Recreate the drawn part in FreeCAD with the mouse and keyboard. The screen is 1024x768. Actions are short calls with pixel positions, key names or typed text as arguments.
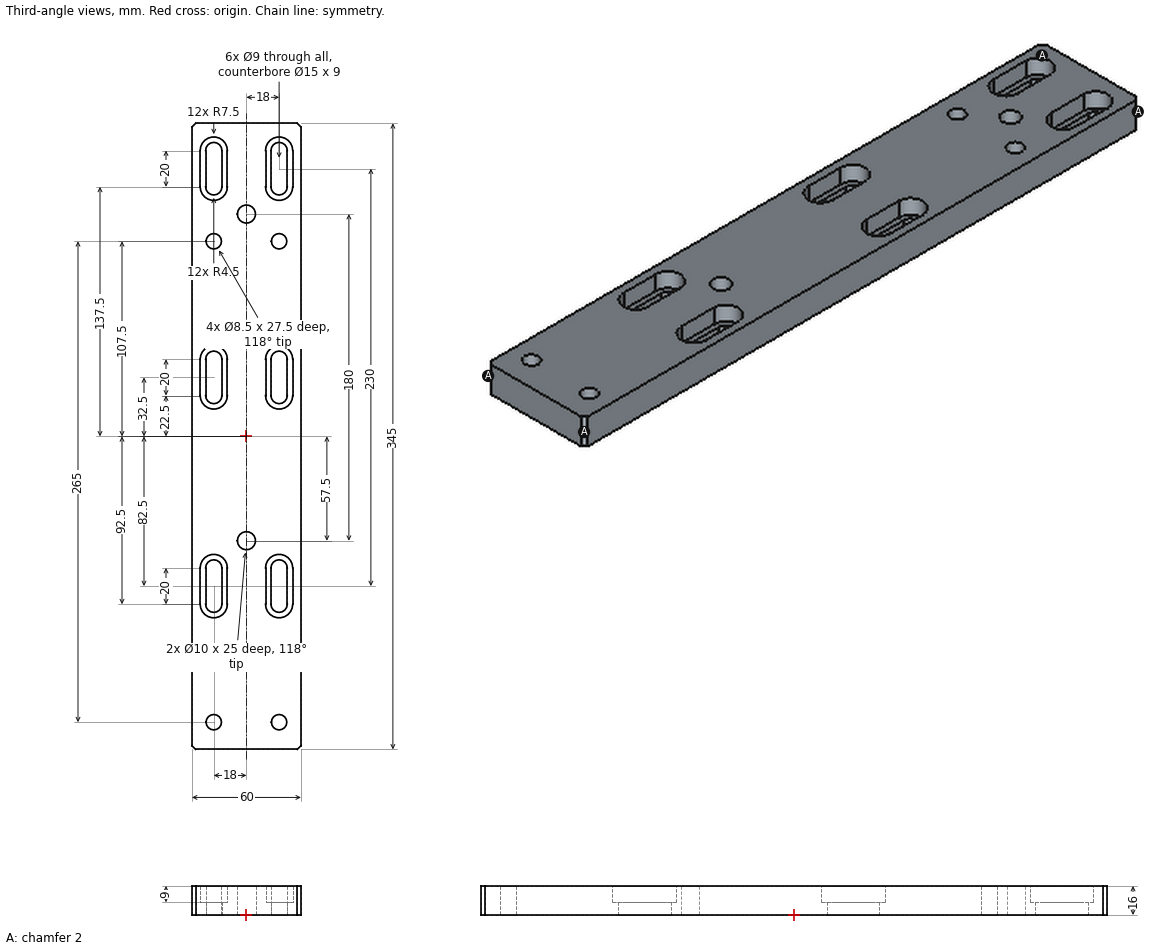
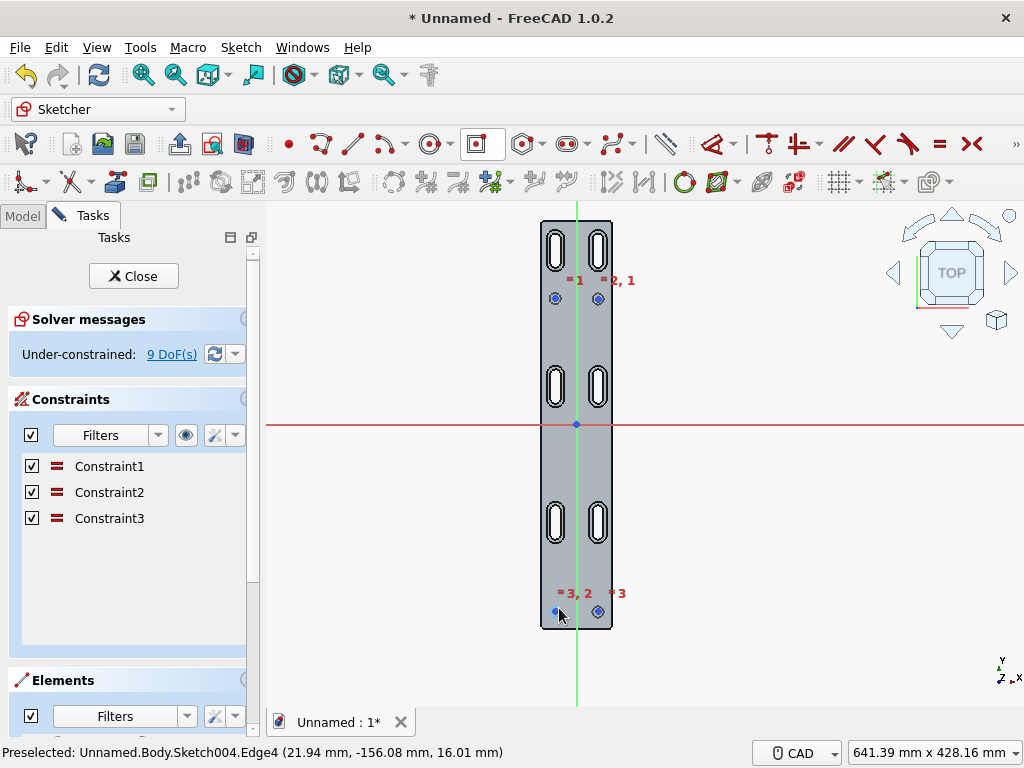
click(555, 299)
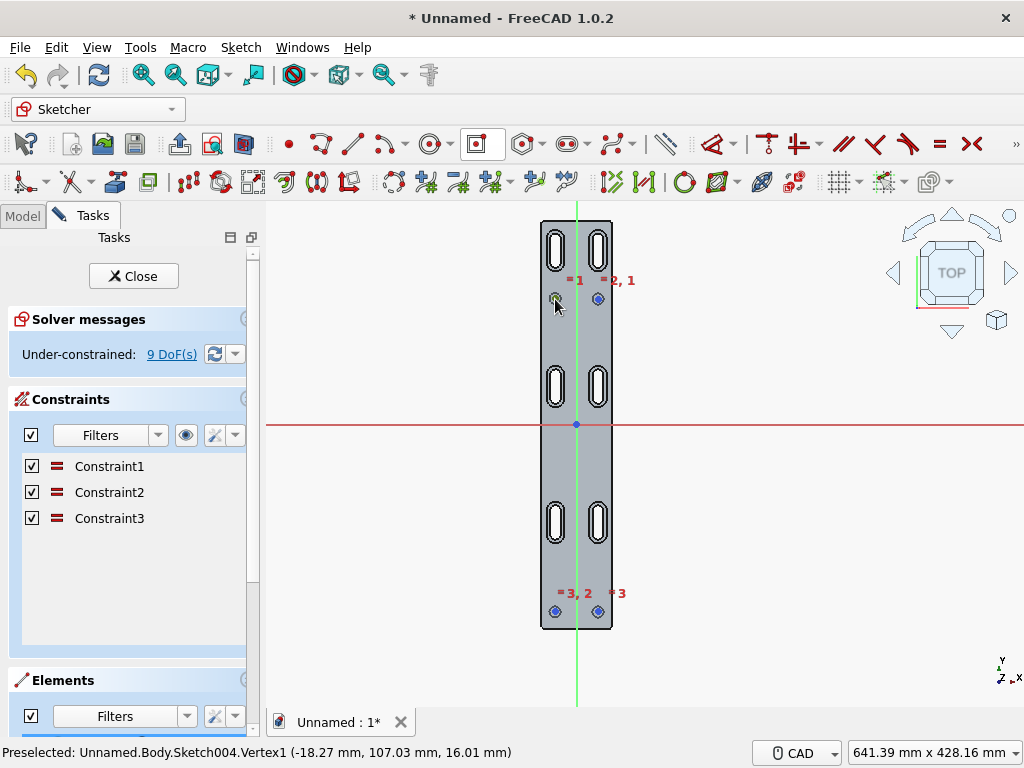
click(598, 299)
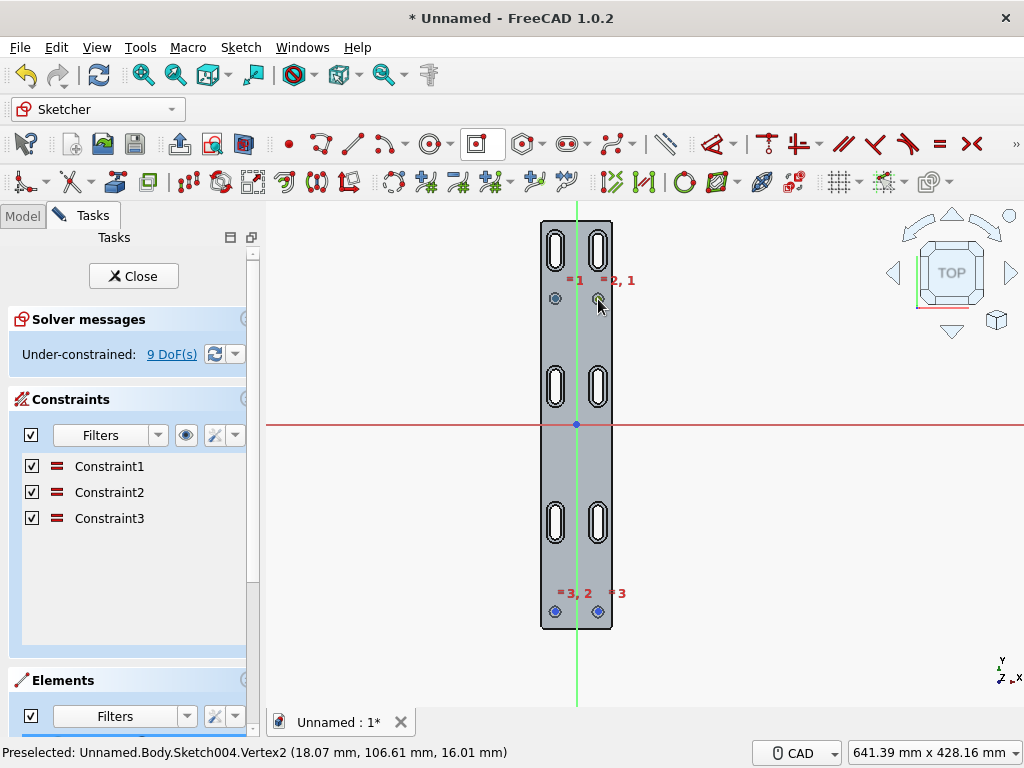
click(577, 647)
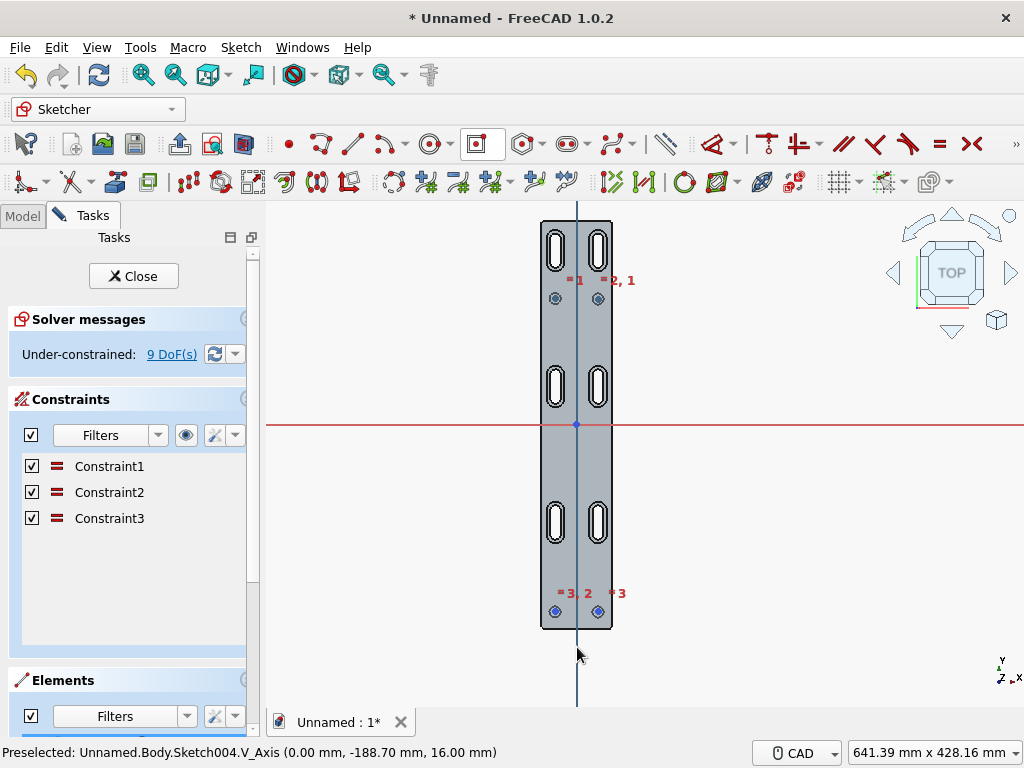
key(s)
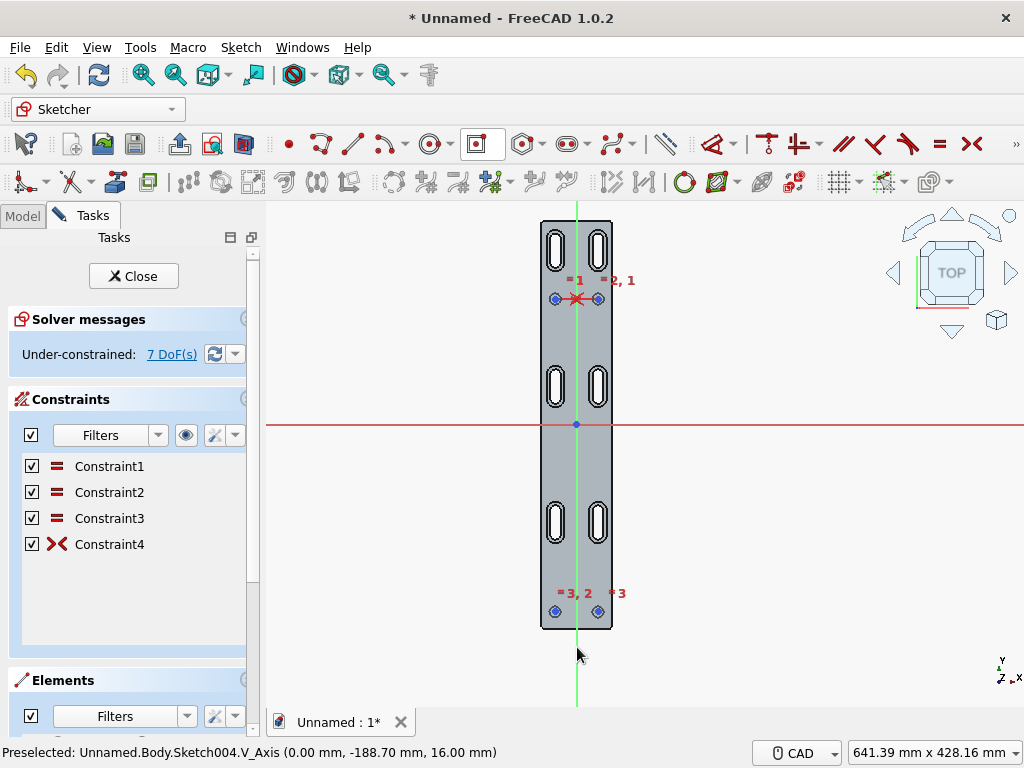
click(555, 612)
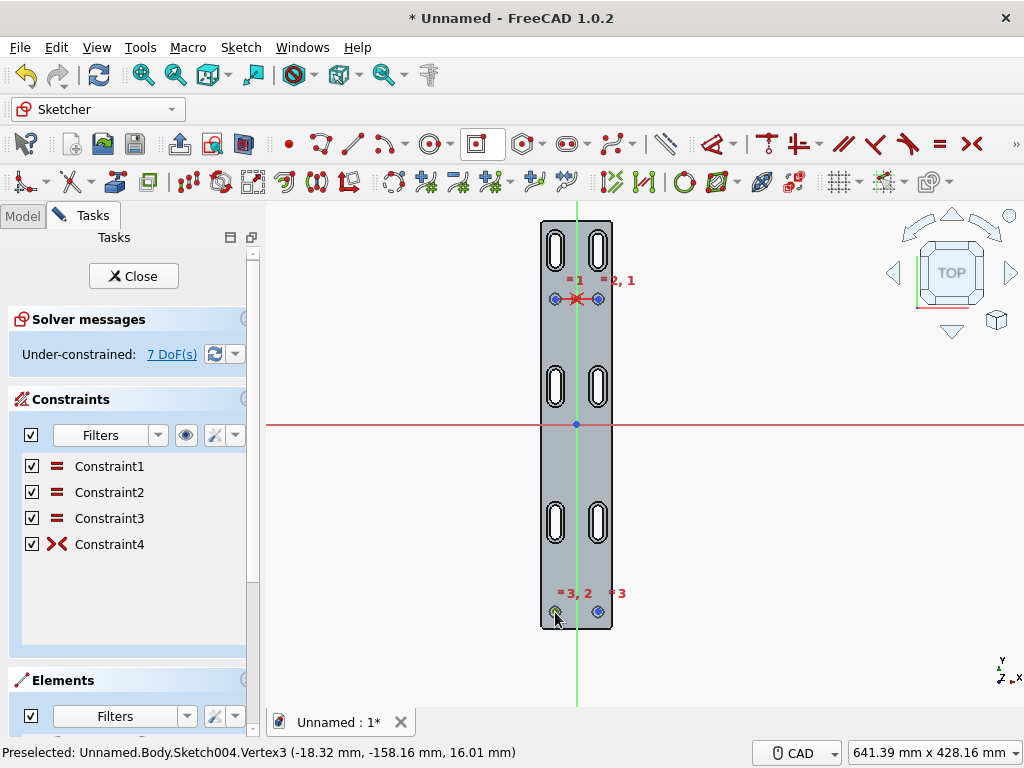
click(598, 612)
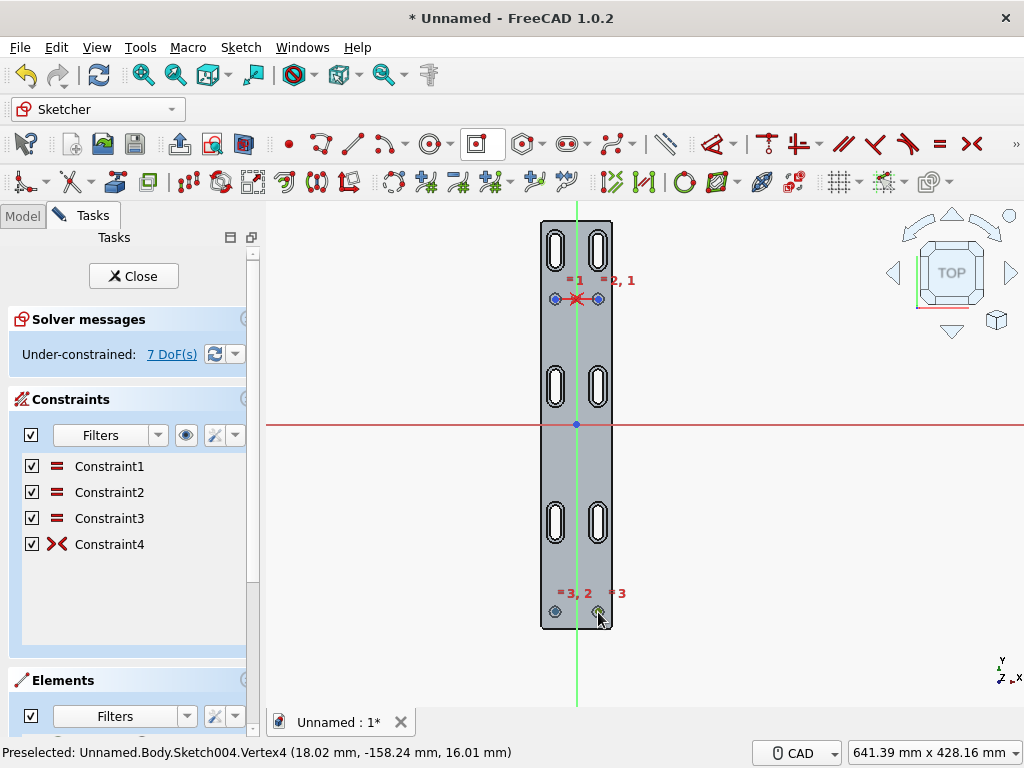
click(577, 647)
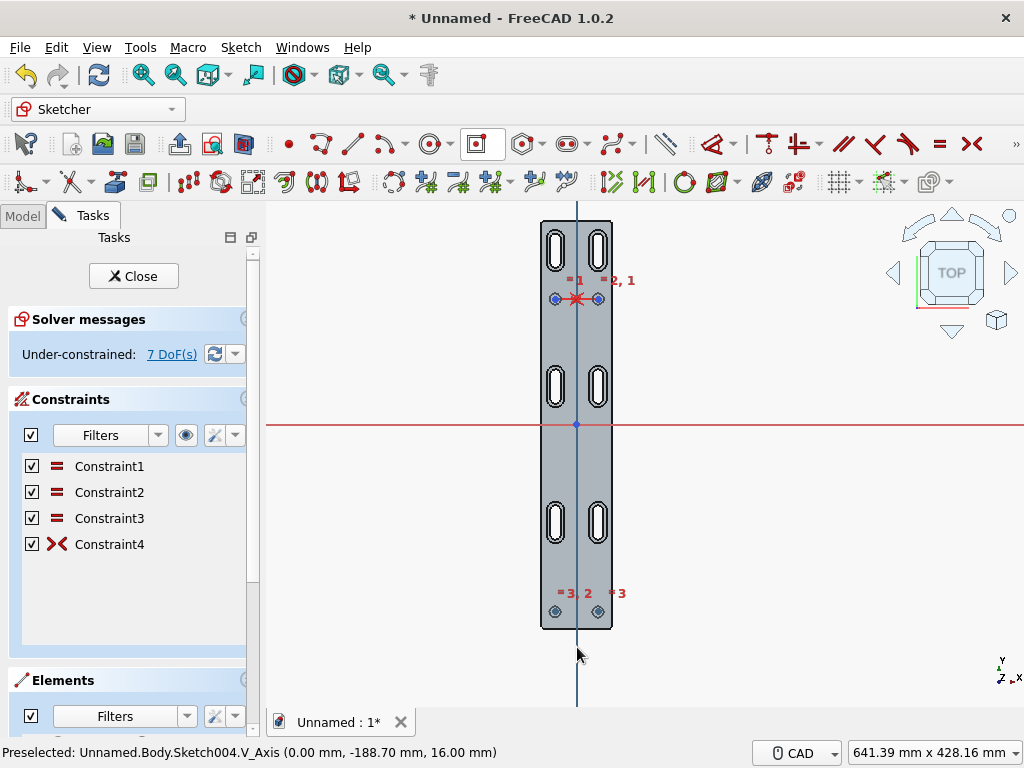
click(972, 144)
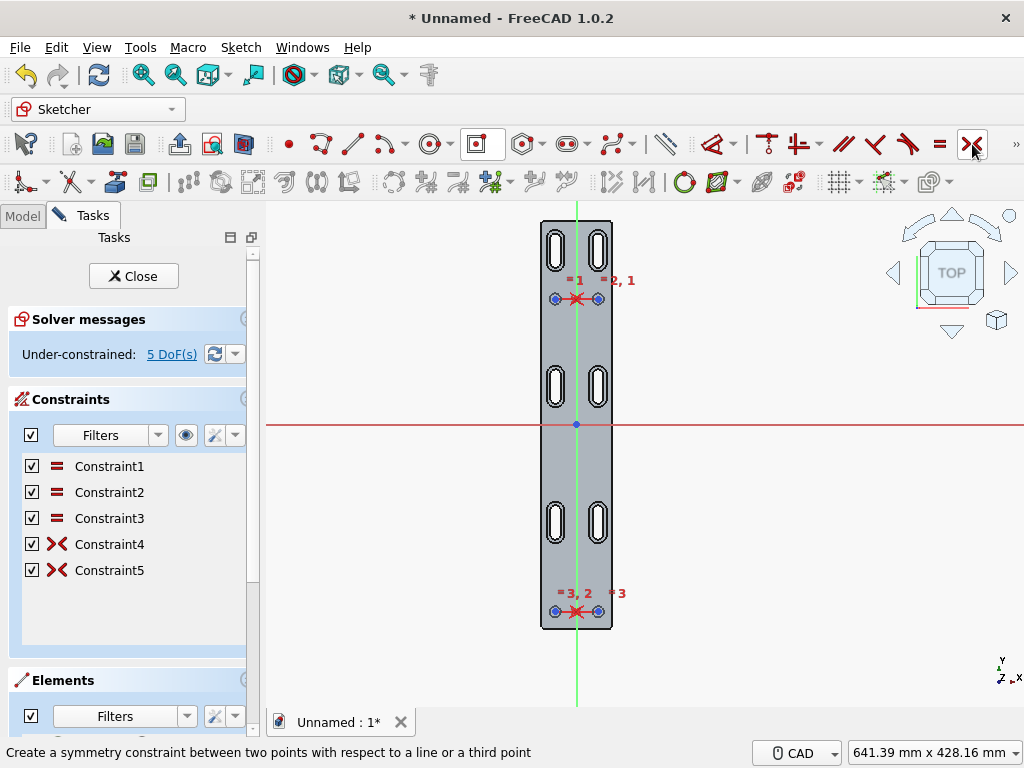
key(d)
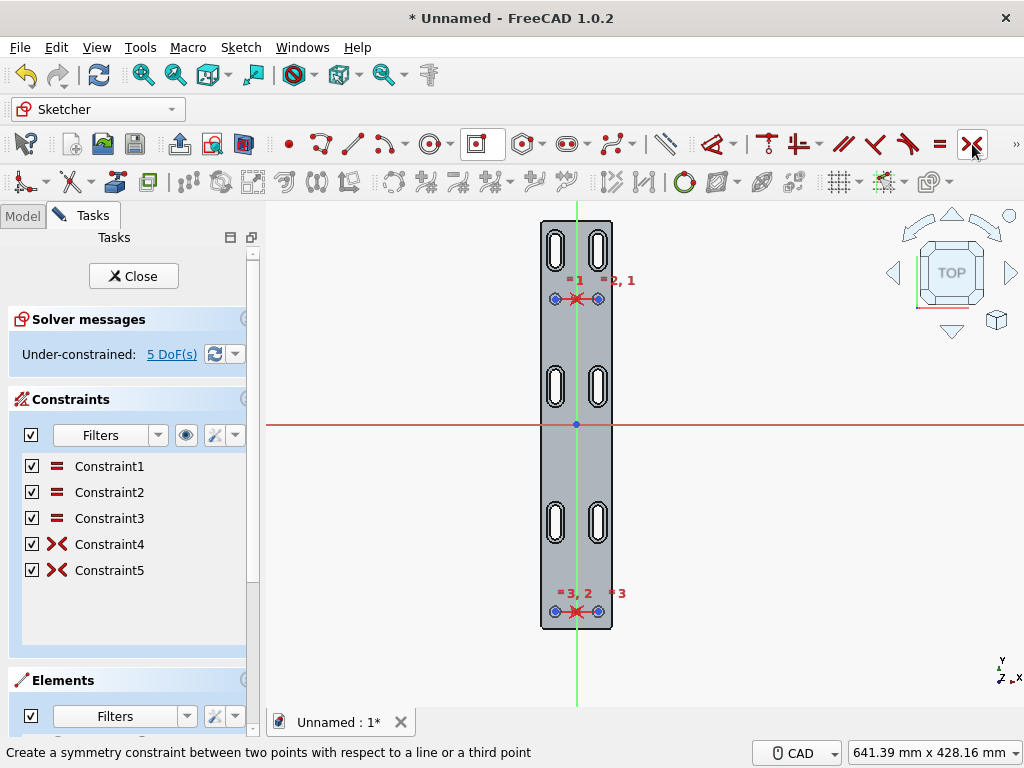
scroll(559, 303, up, 7)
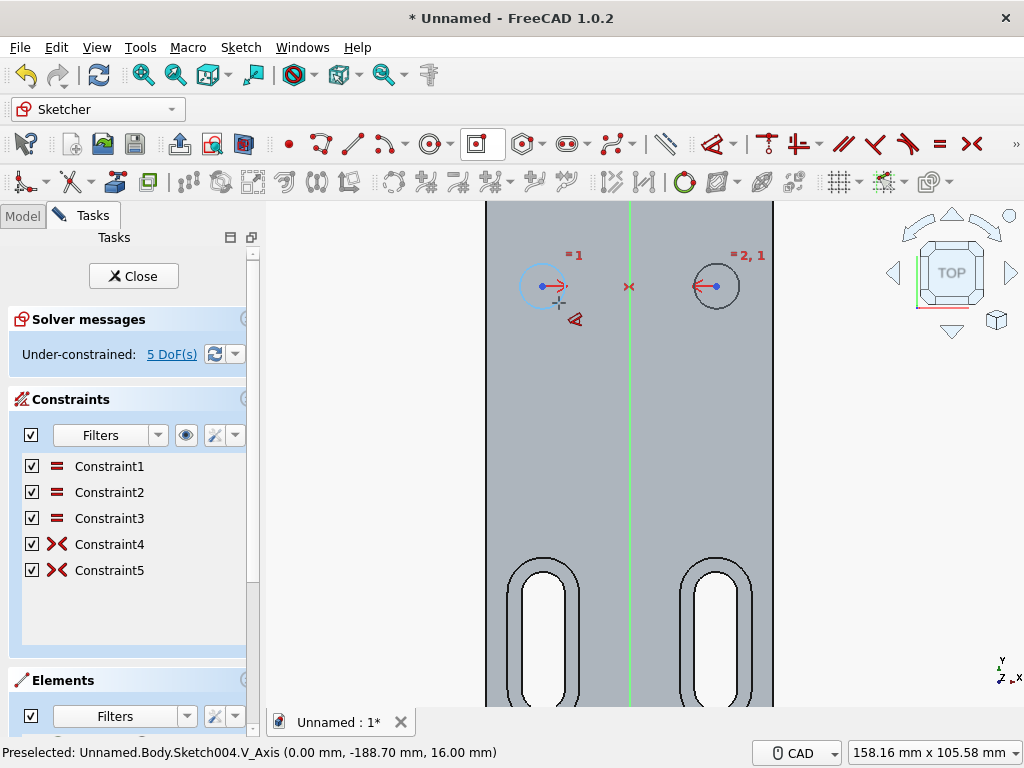
click(558, 302)
click(580, 325)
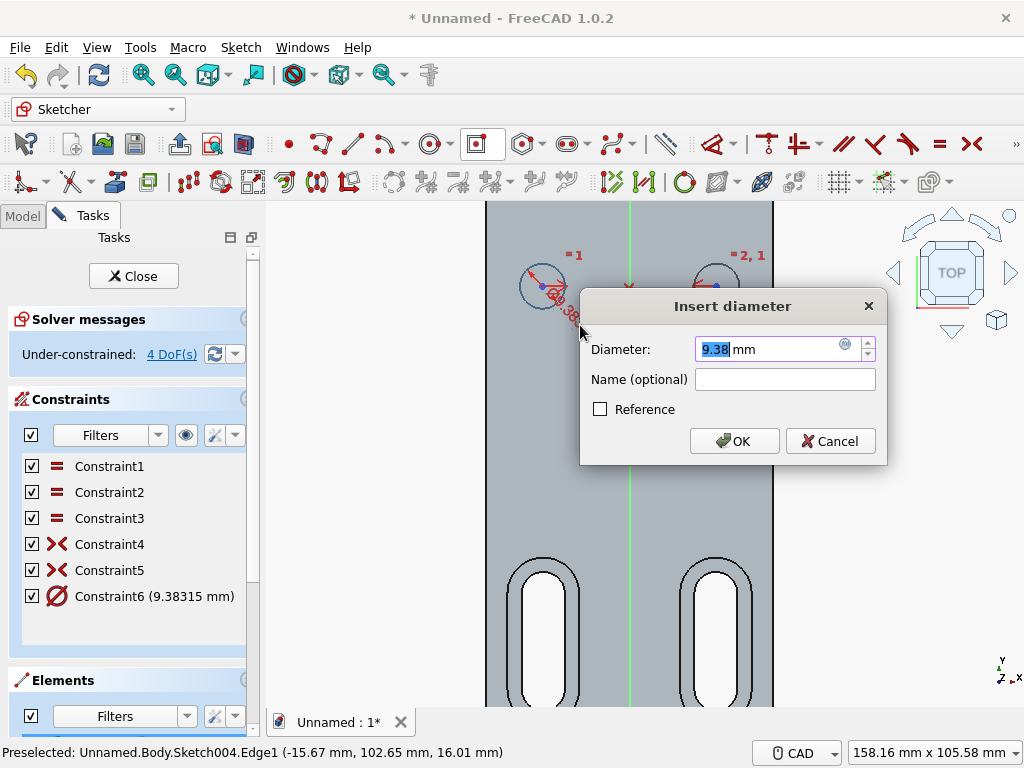
text(8.5)
key(Return)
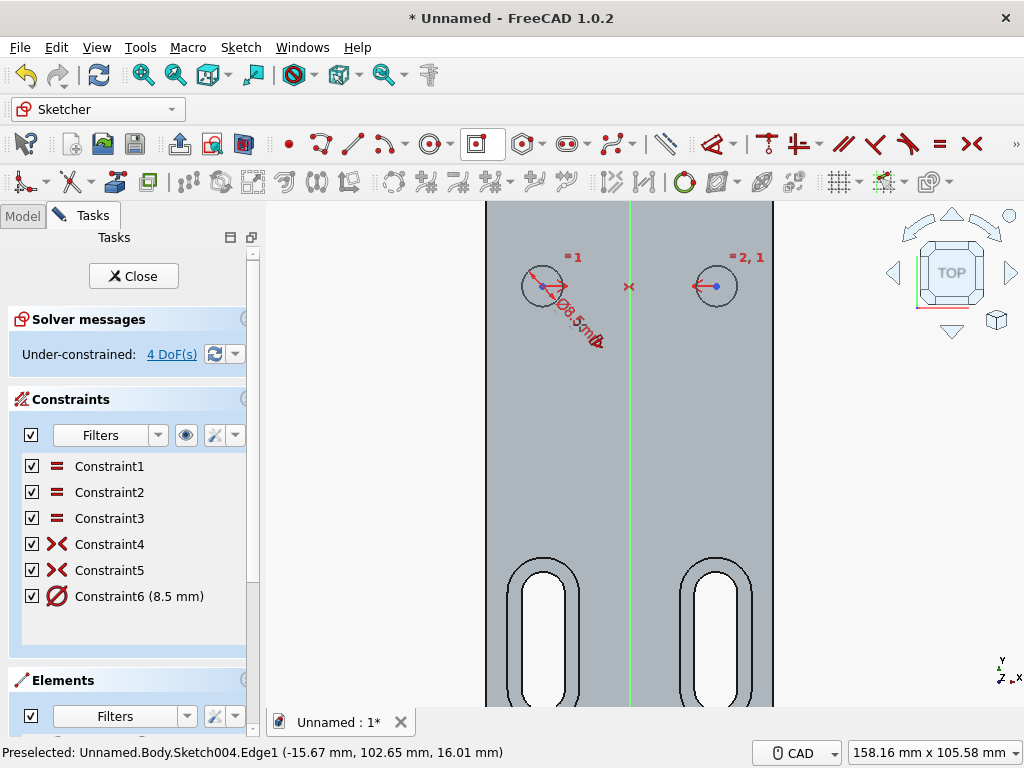
click(542, 286)
click(586, 252)